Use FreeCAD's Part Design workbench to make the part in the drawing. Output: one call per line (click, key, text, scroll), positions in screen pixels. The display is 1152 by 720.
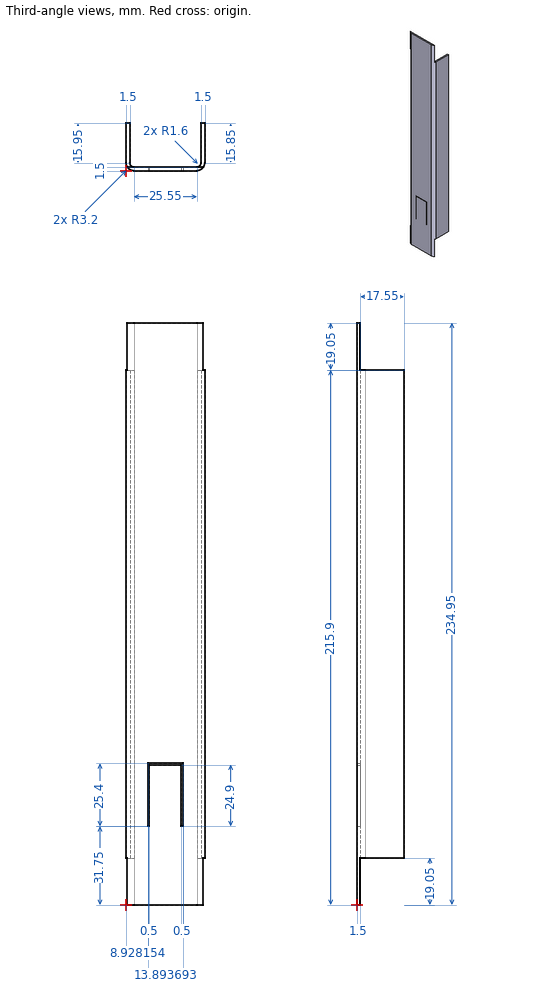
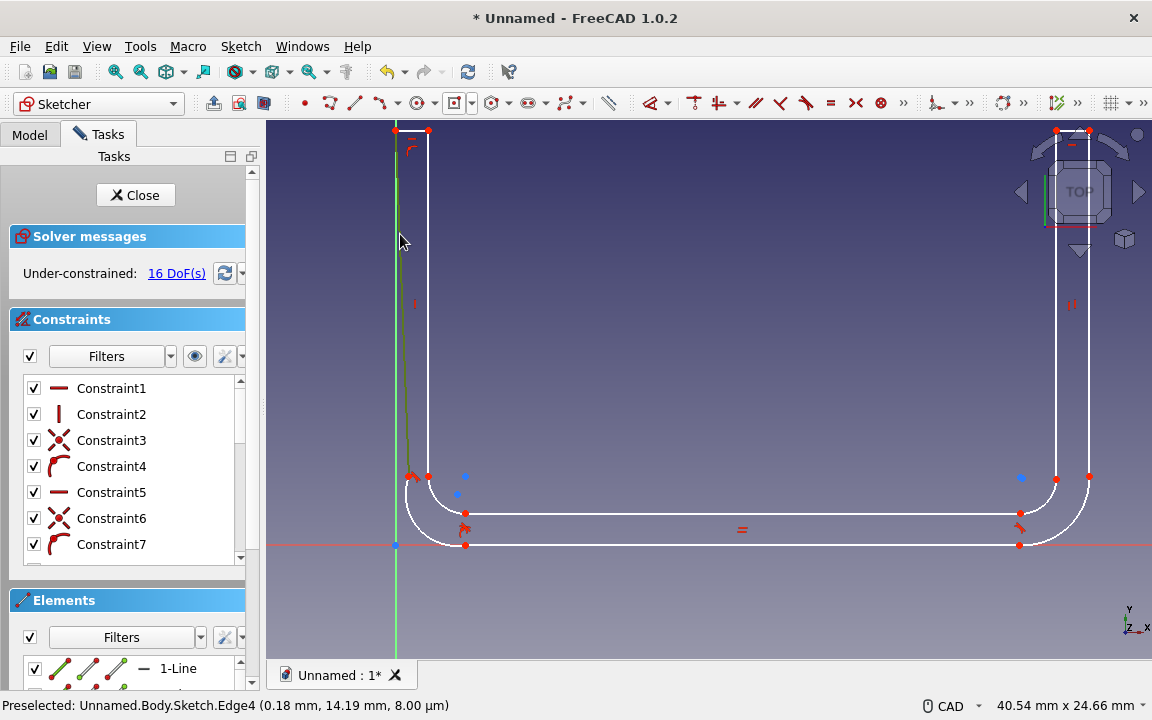
click(408, 508)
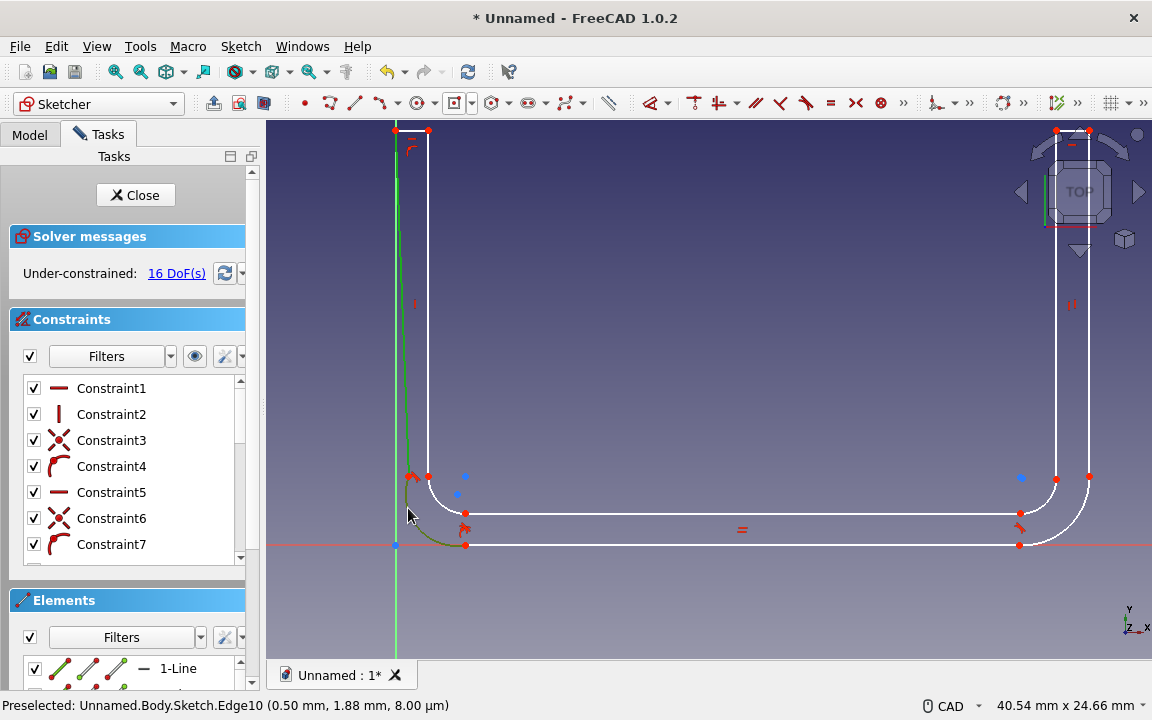
click(806, 104)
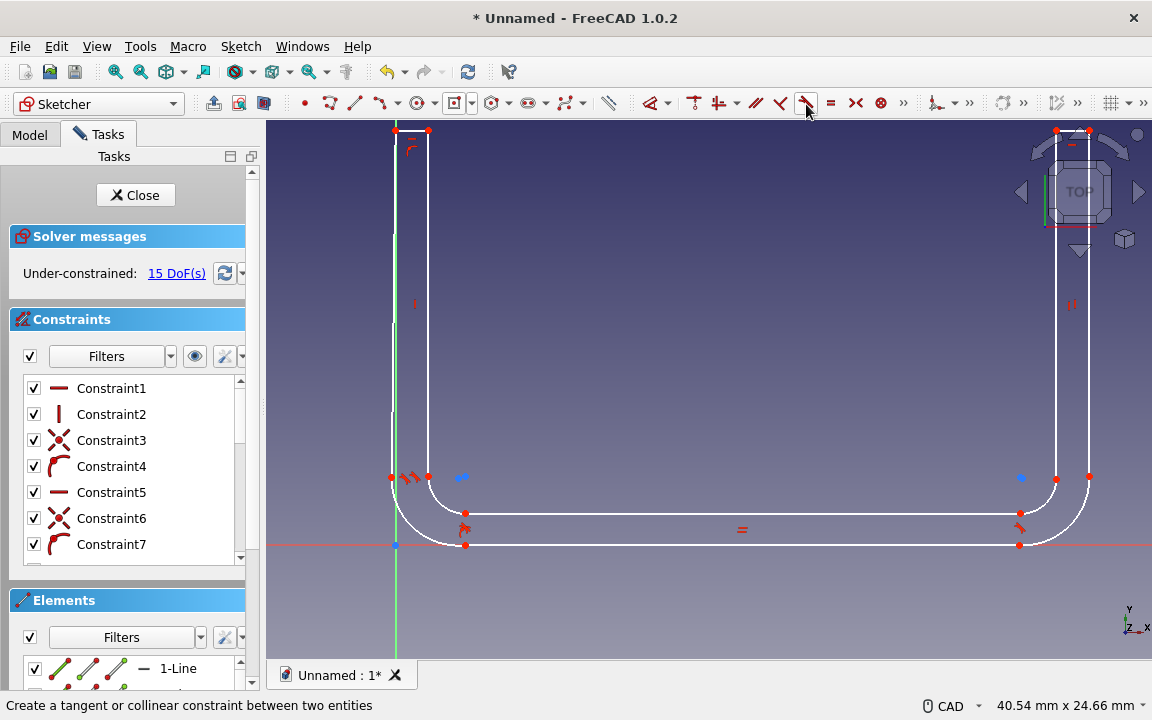
click(632, 545)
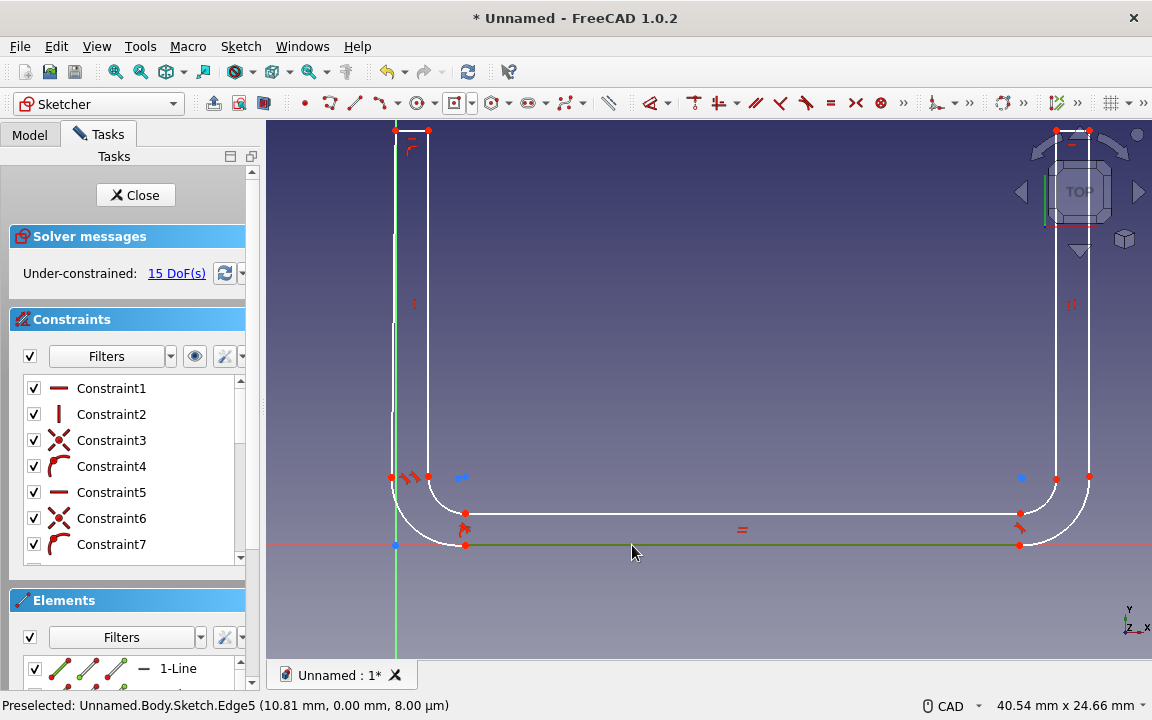
click(414, 528)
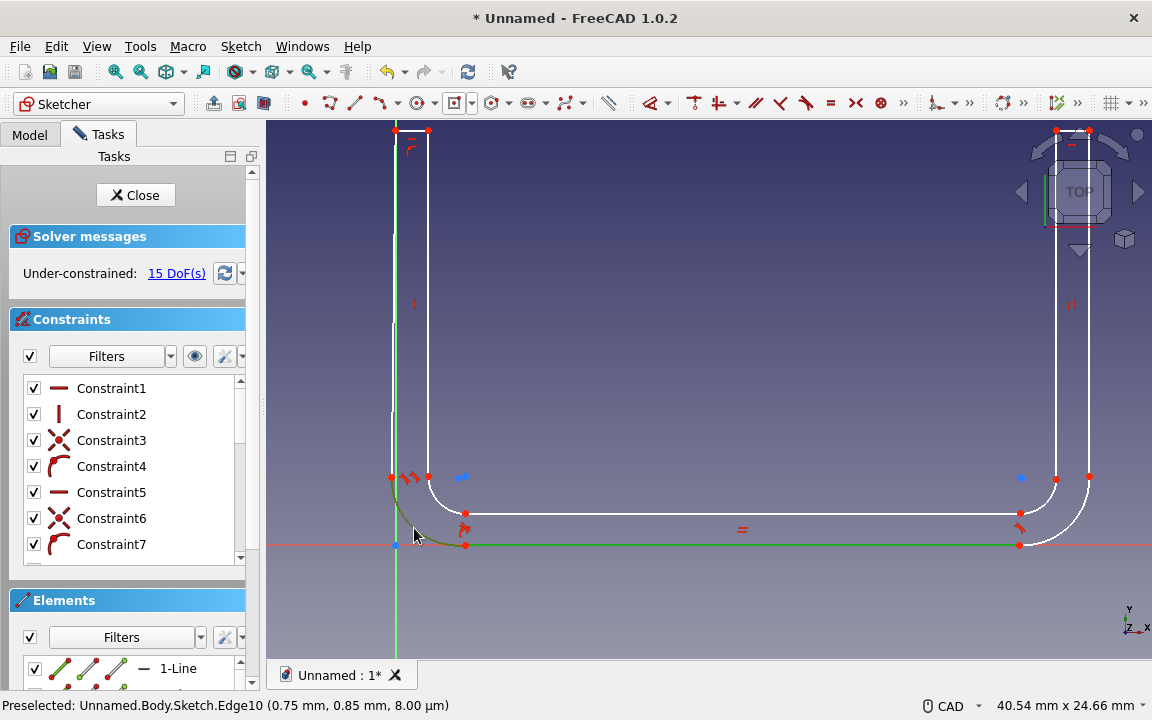
key(t)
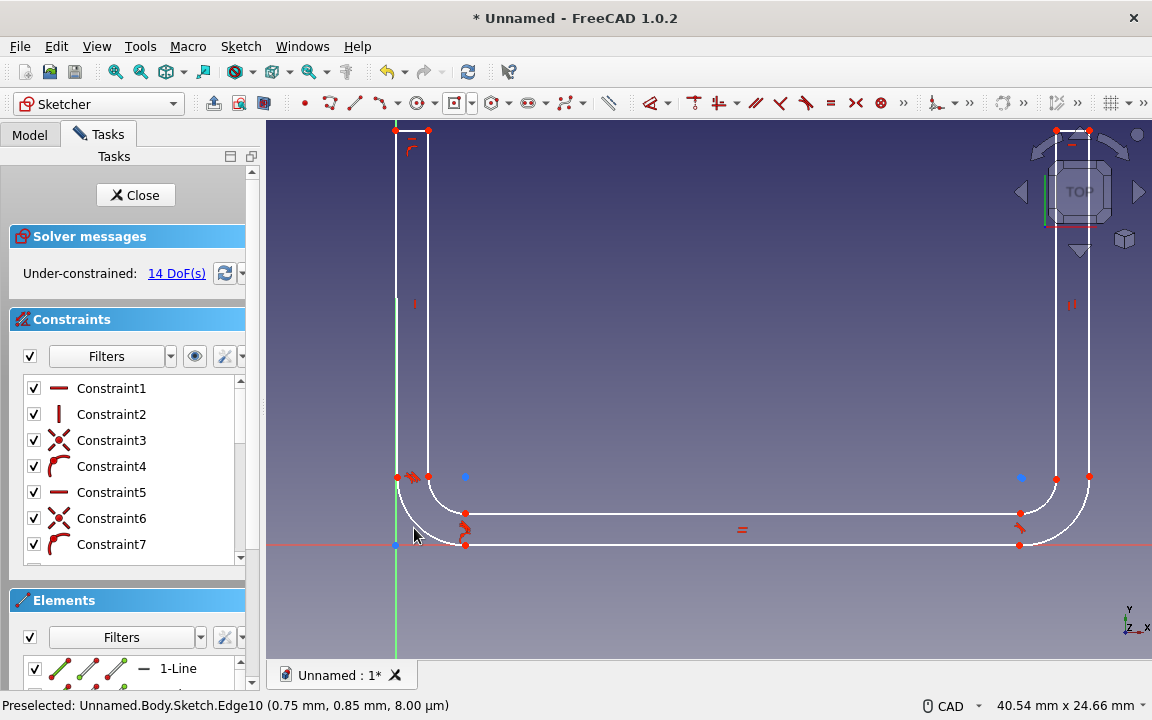
click(632, 545)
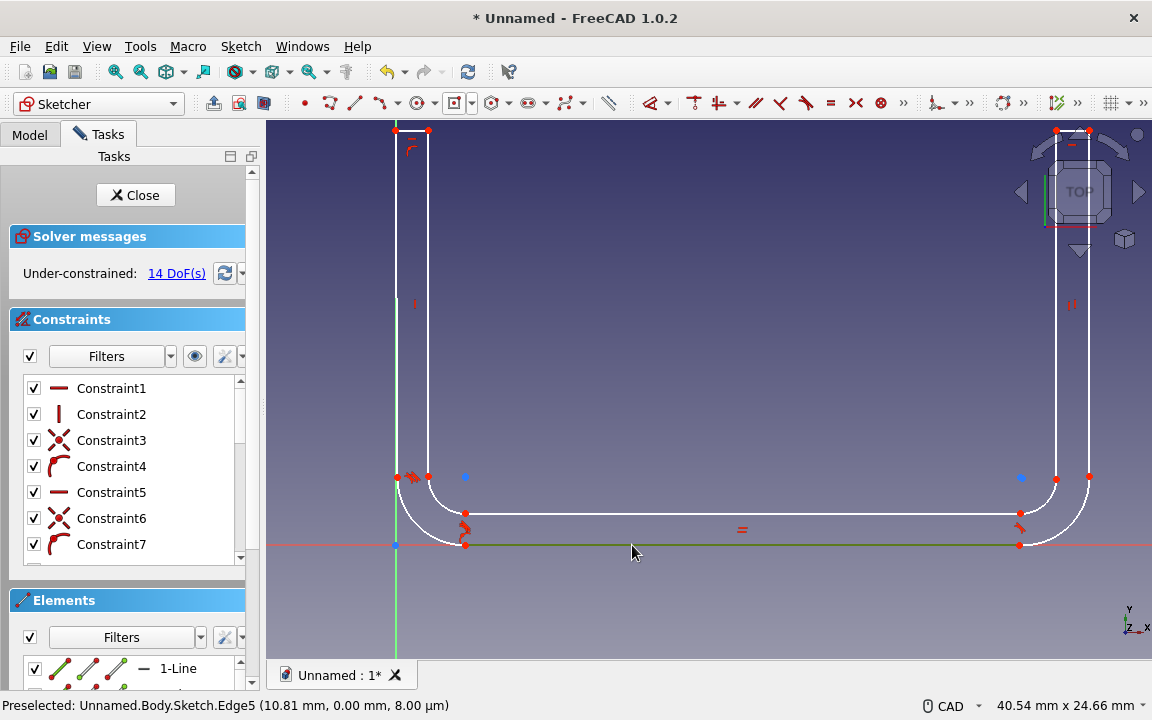
scroll(433, 496, down, 2)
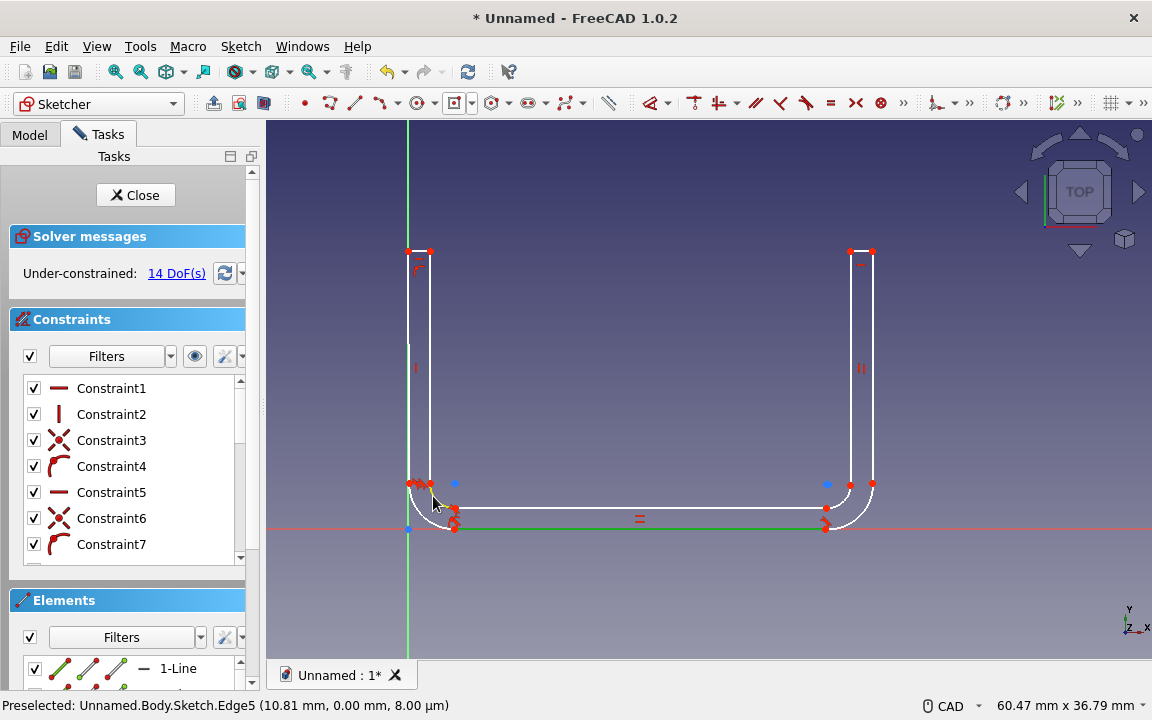
click(868, 505)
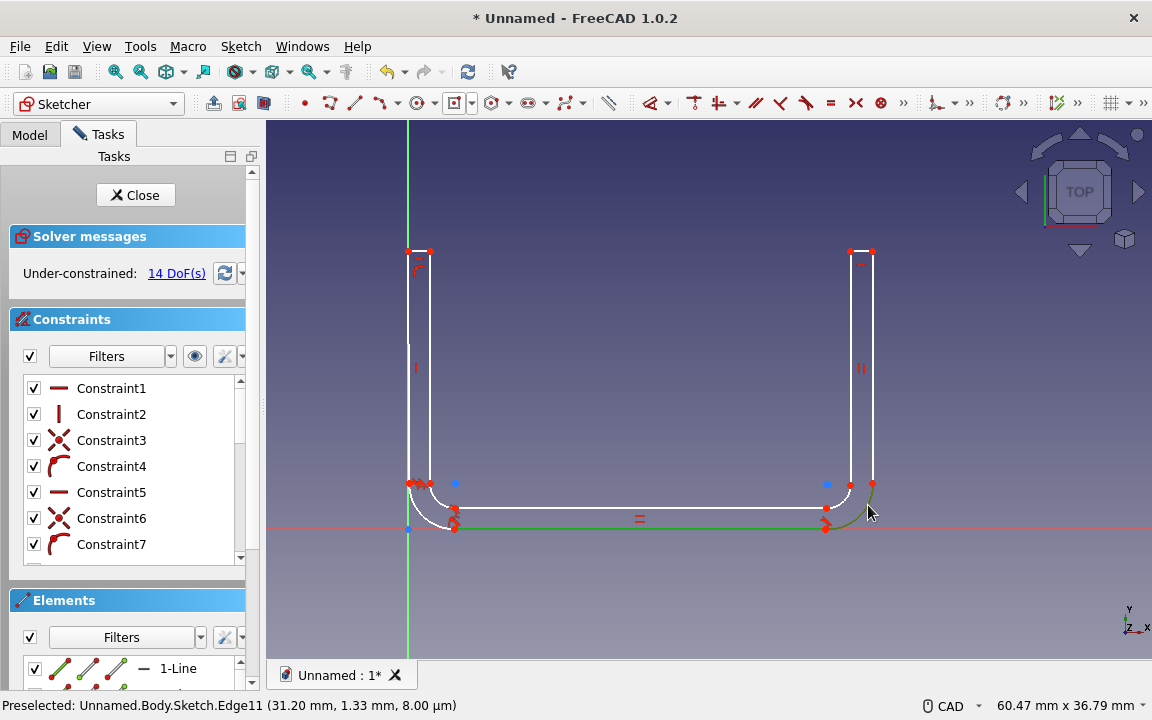
key(t)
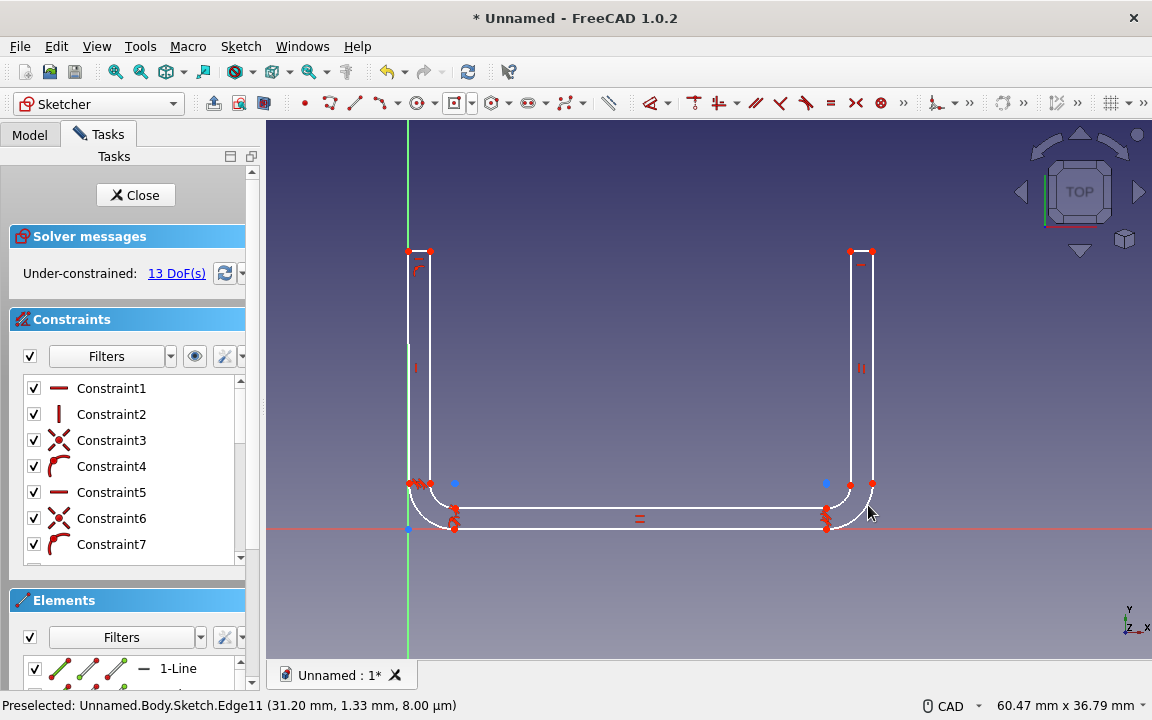
click(873, 414)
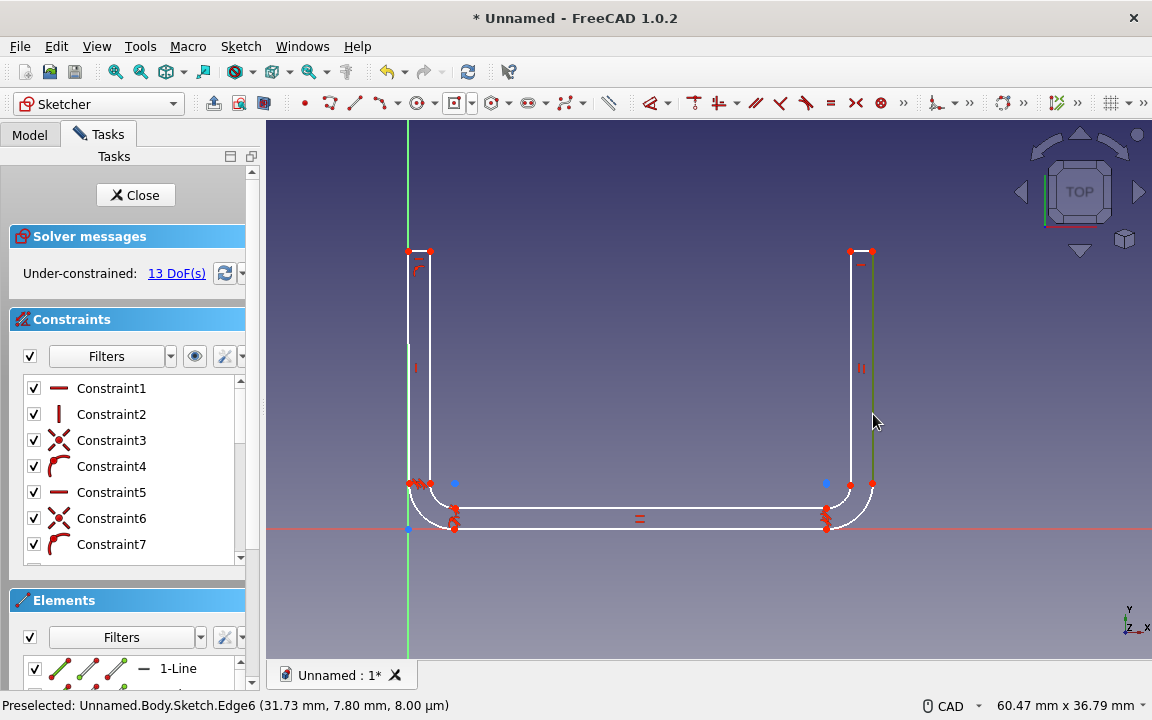
click(868, 504)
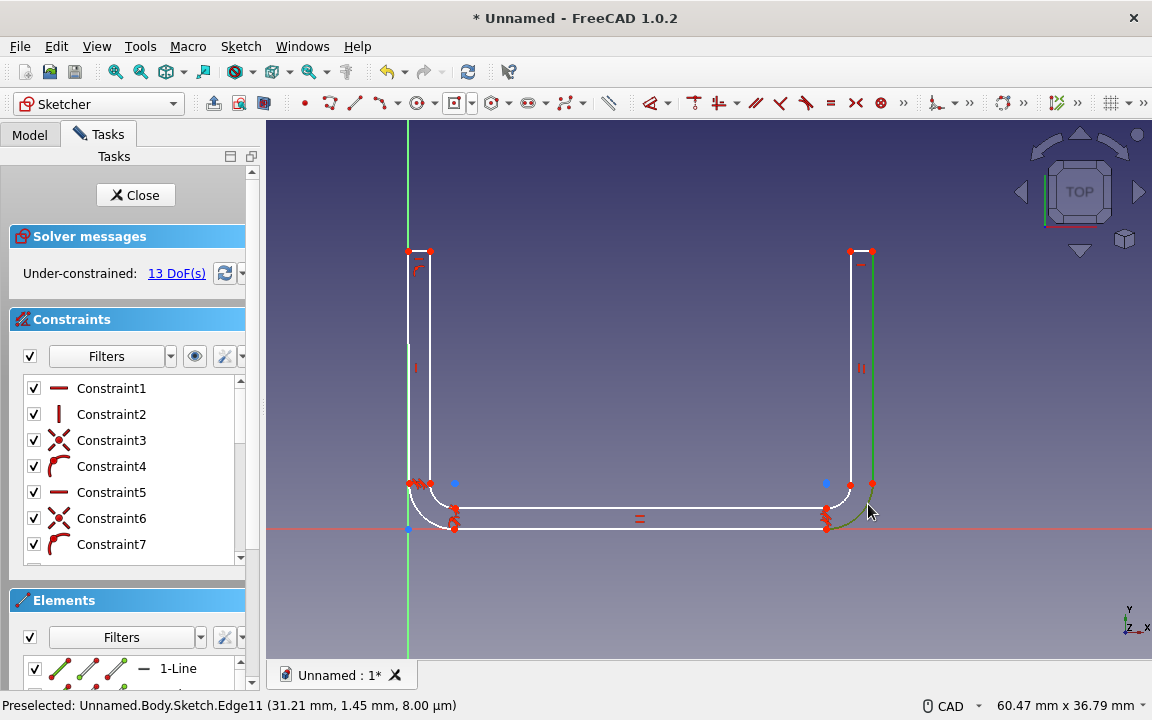
click(806, 104)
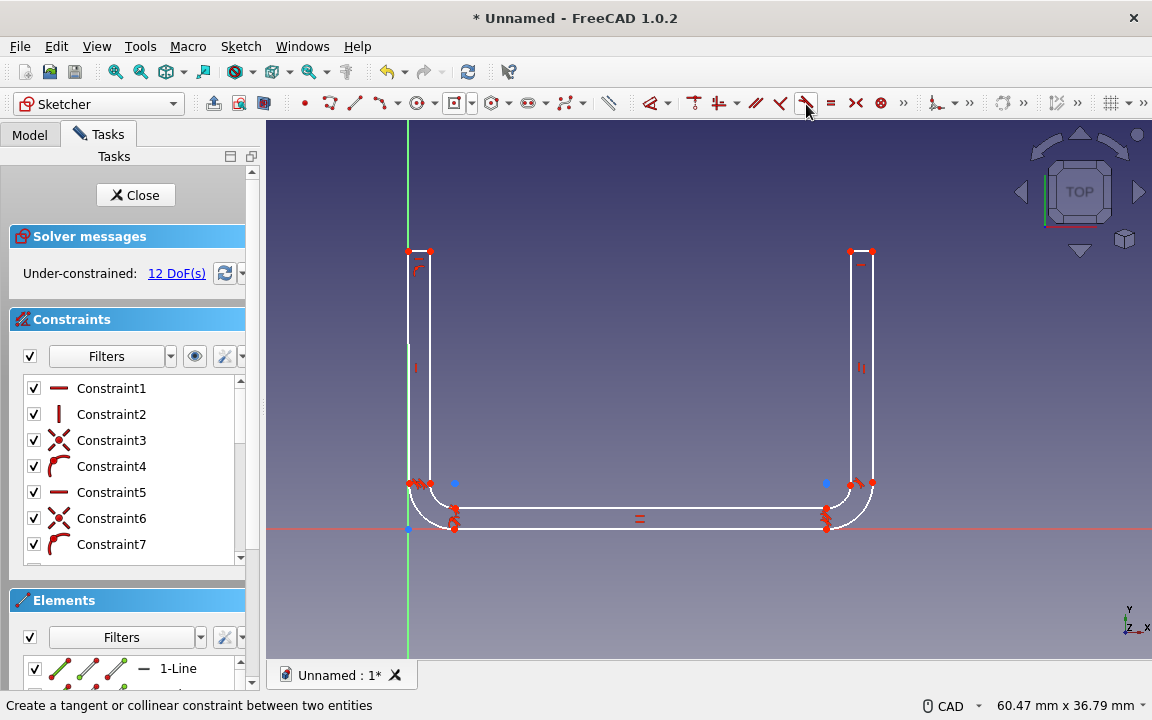
click(851, 322)